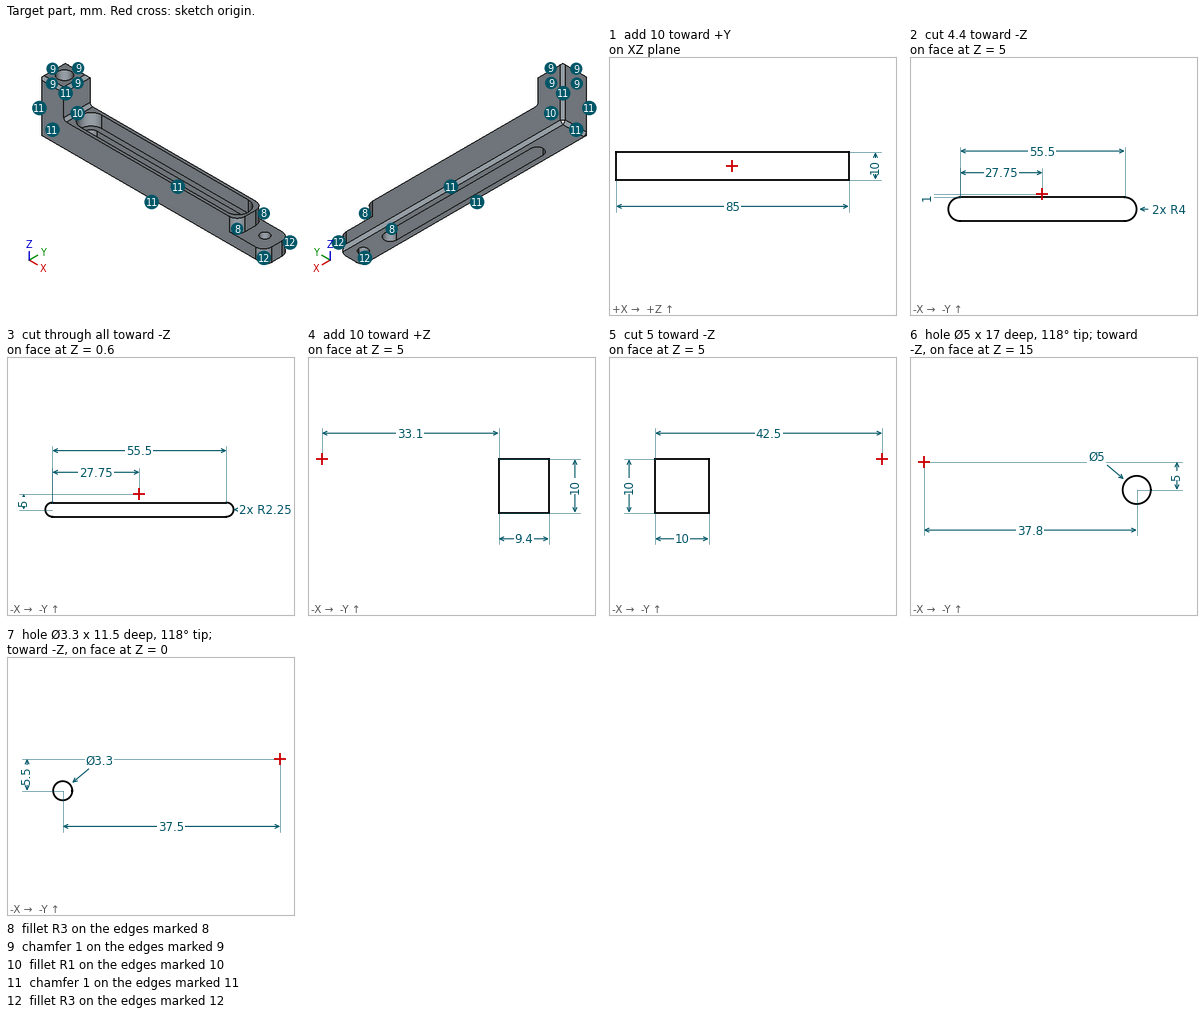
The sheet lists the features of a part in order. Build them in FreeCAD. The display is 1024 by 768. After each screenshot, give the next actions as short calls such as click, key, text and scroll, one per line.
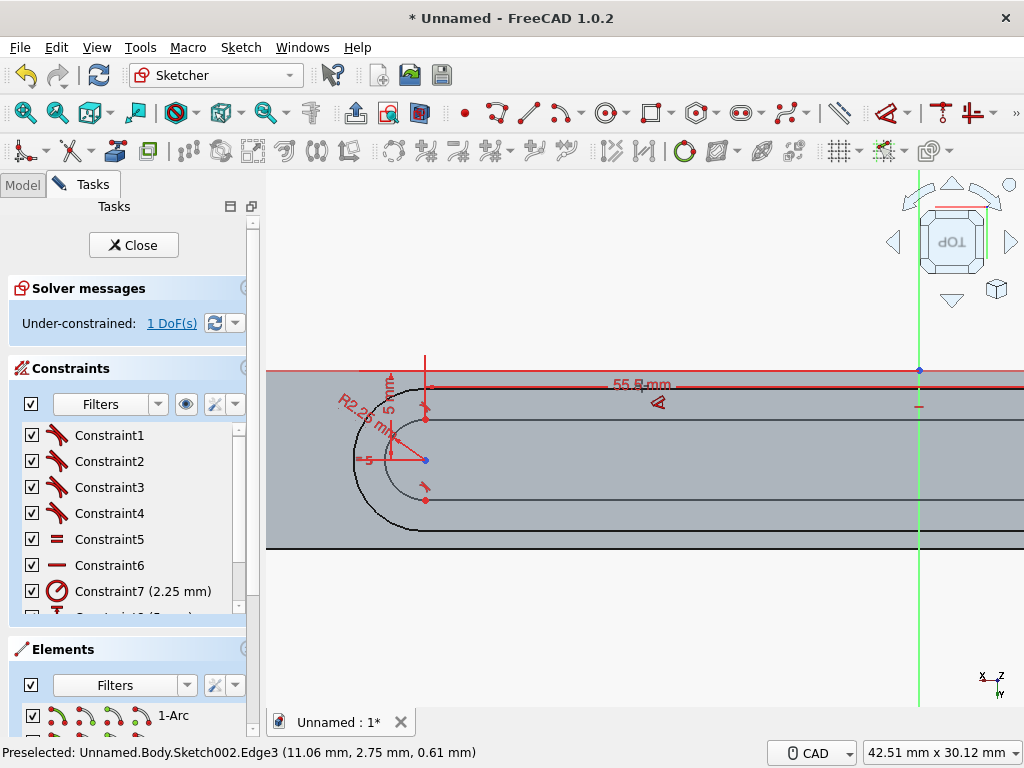
click(425, 420)
click(642, 337)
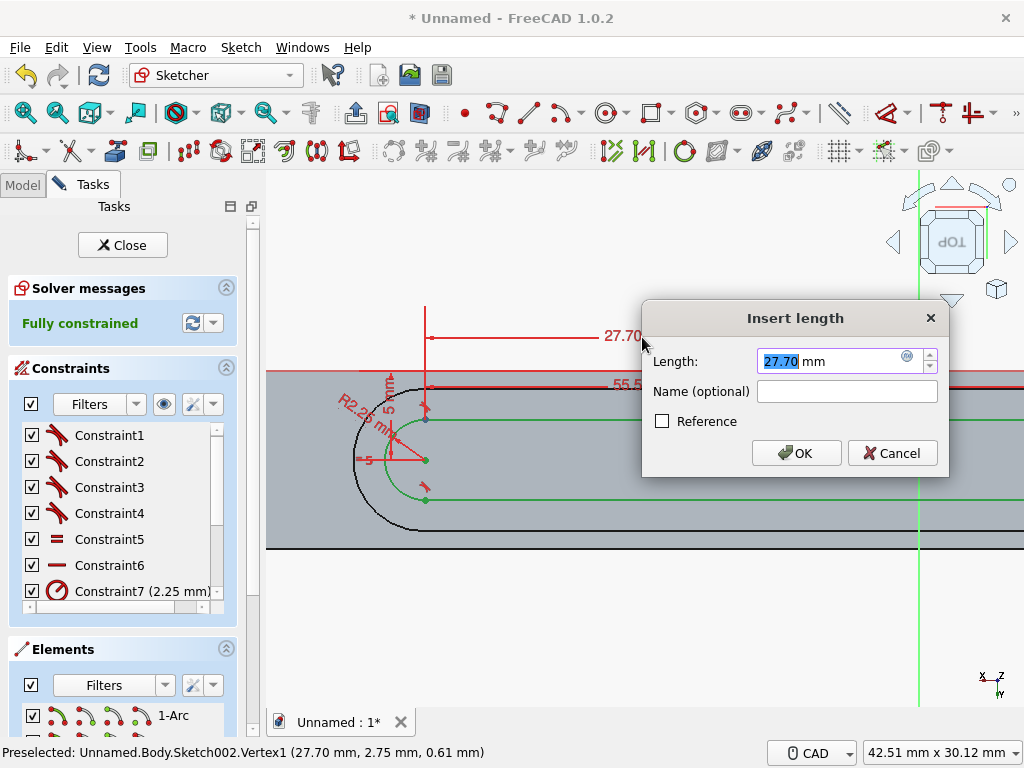
text(27.75)
key(Return)
key(Escape)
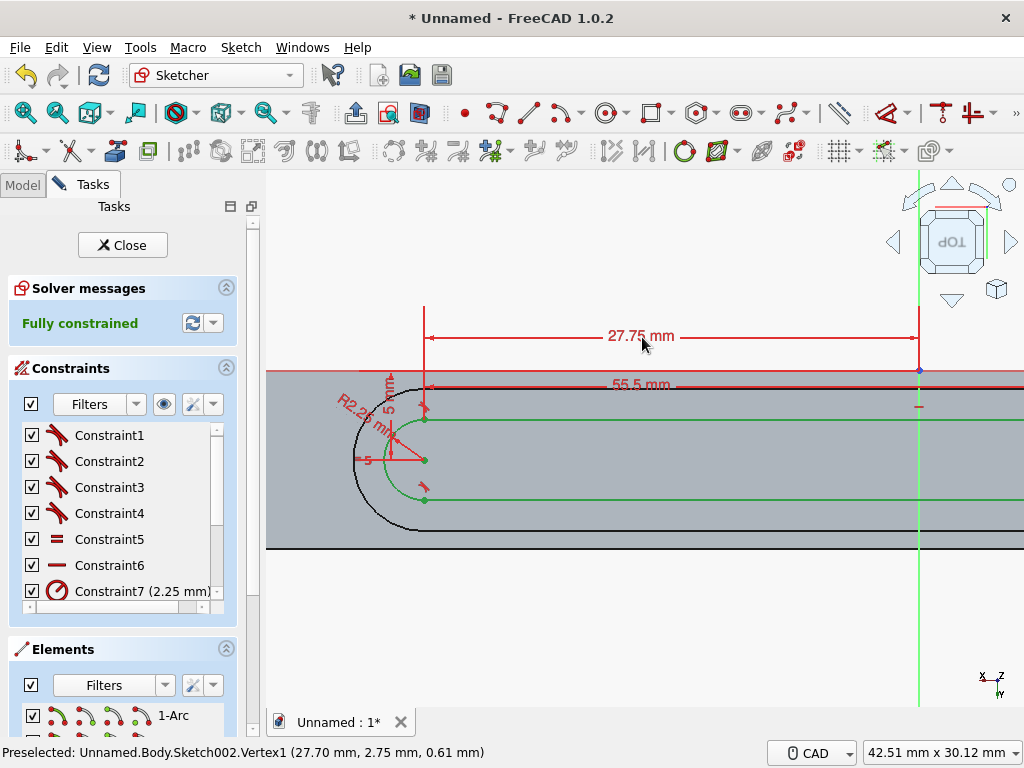
click(123, 245)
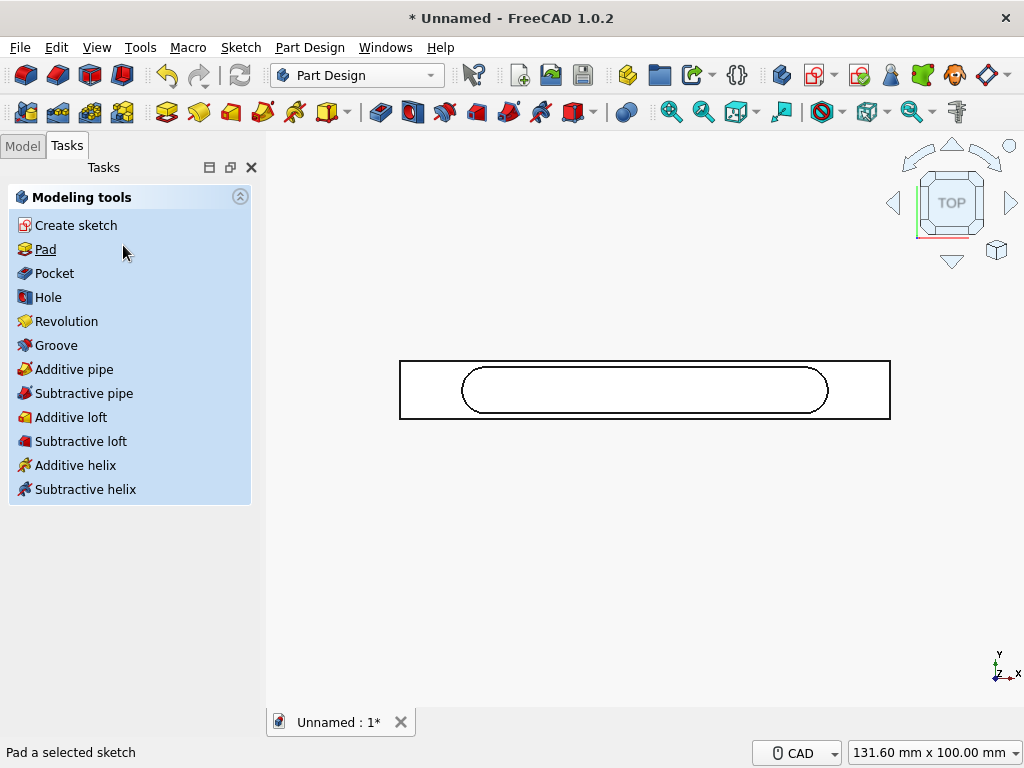
click(382, 112)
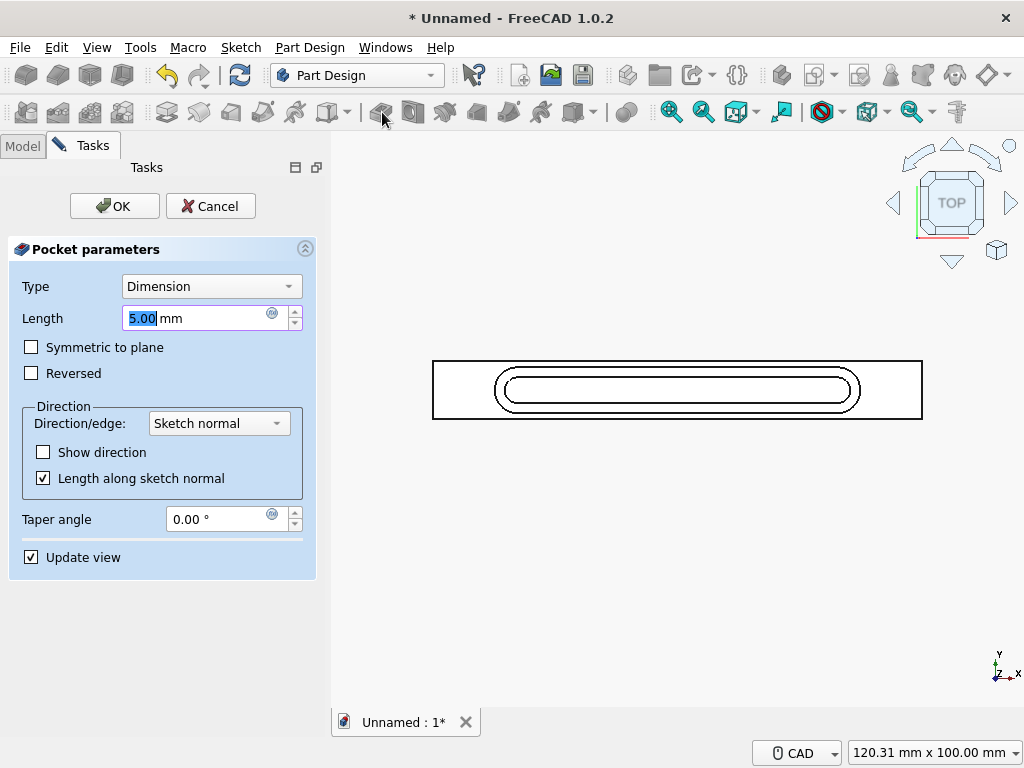
click(212, 286)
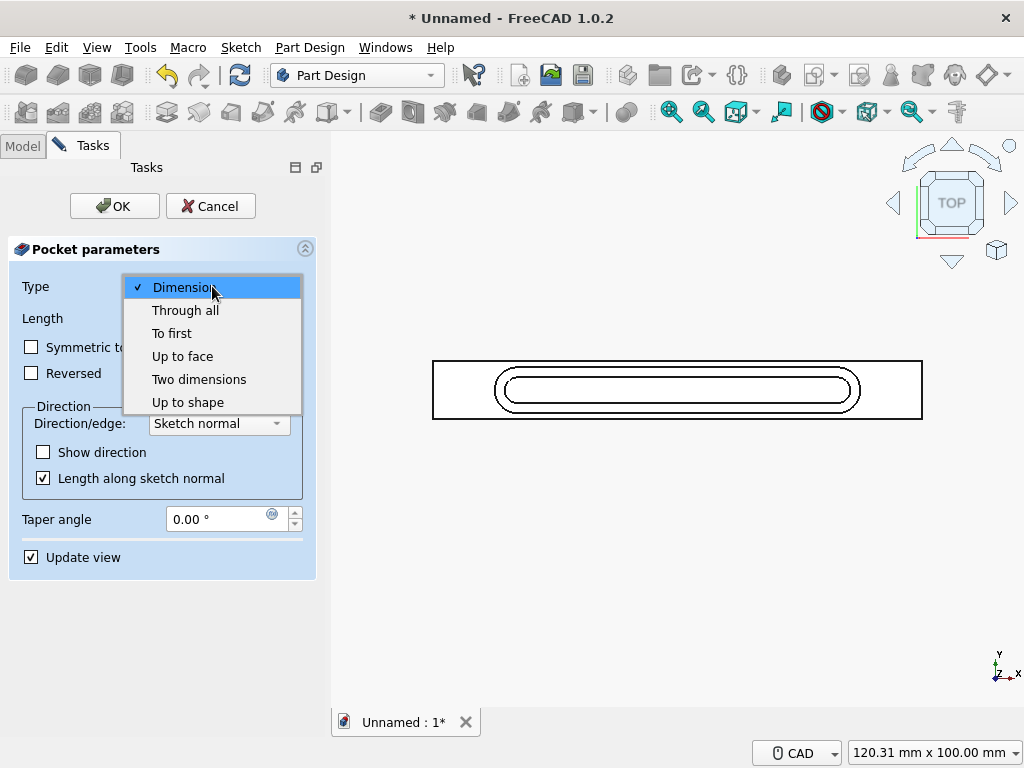
click(212, 310)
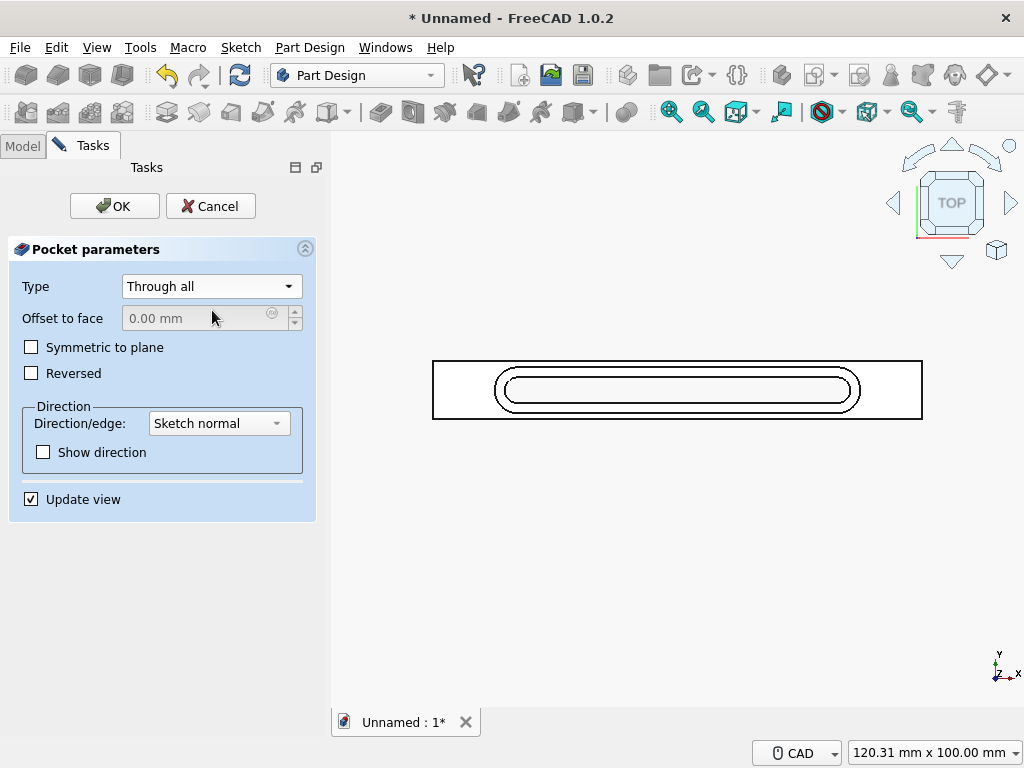
click(115, 206)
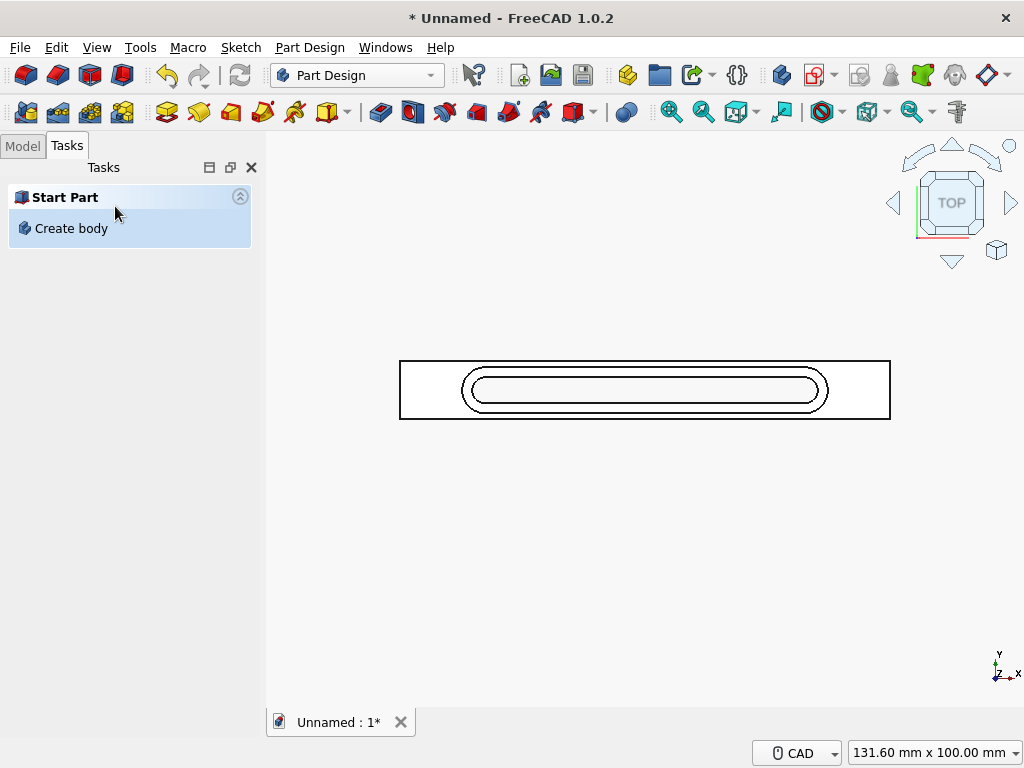
click(855, 389)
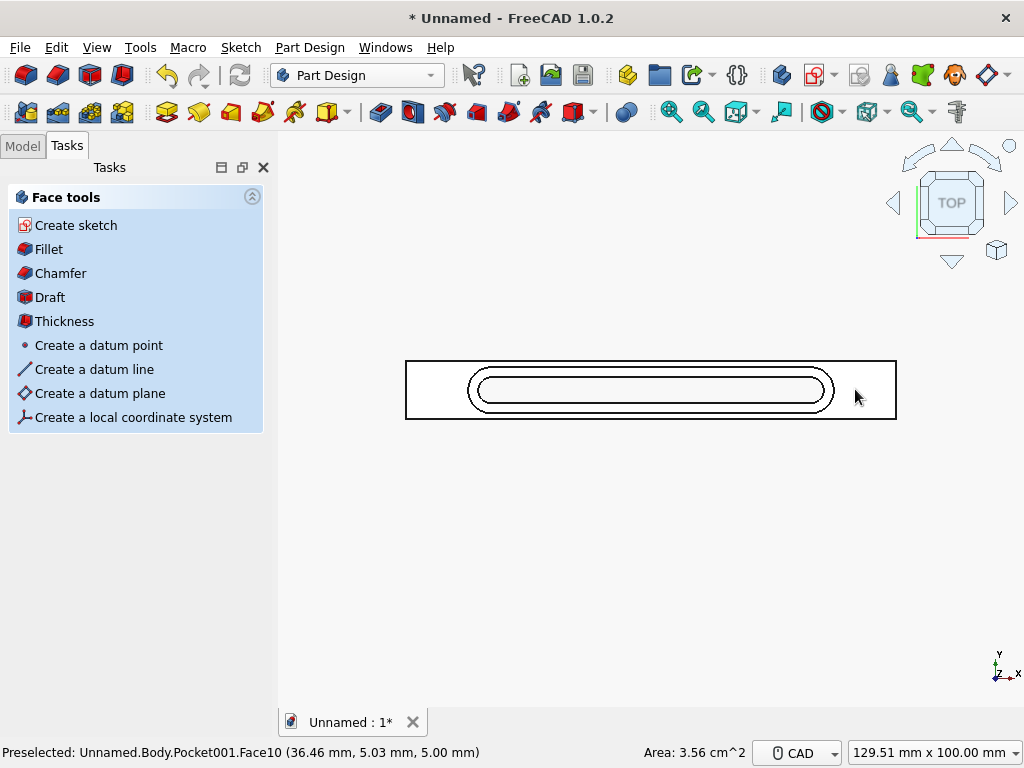
click(814, 76)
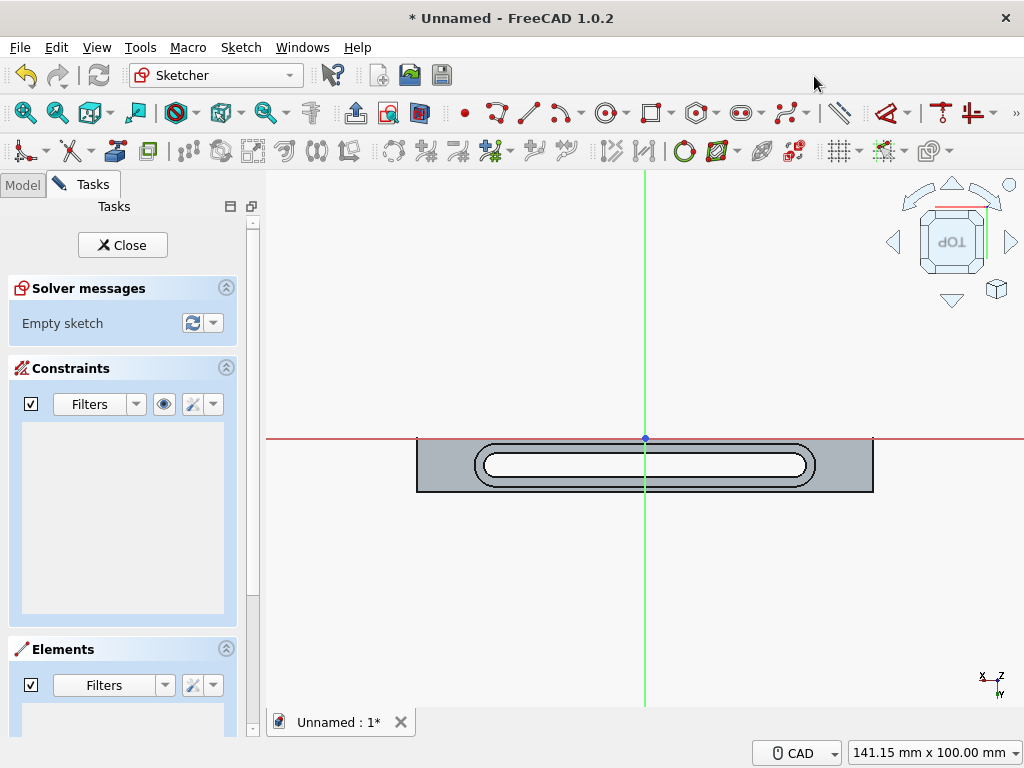
scroll(576, 438, down, 5)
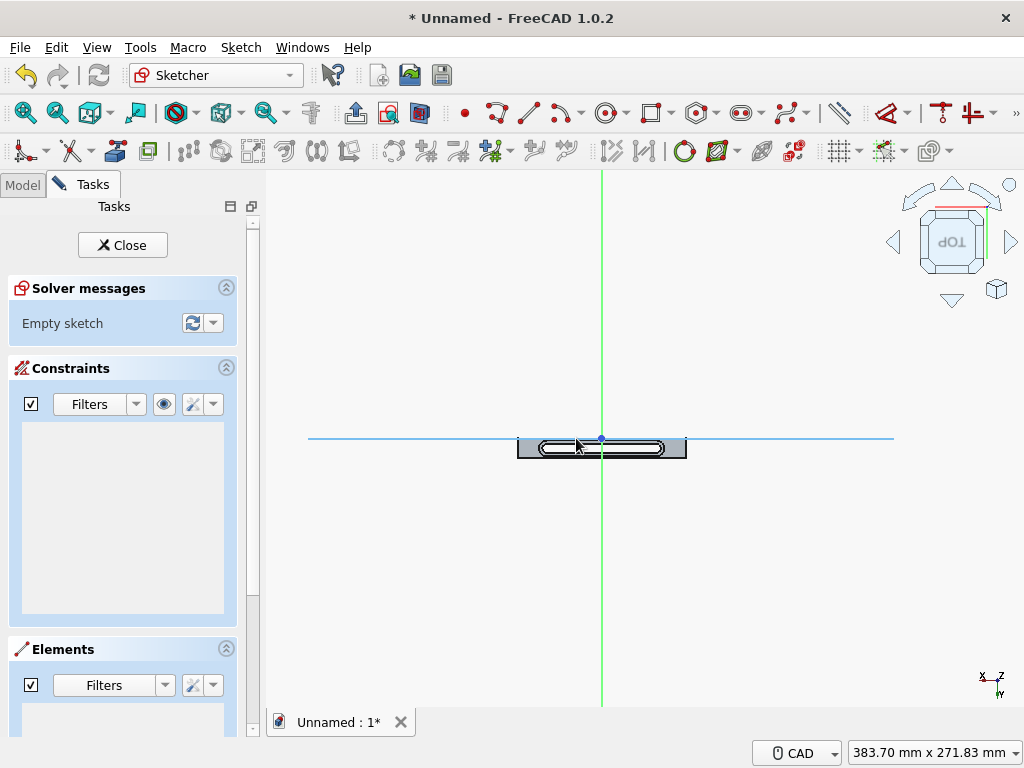
scroll(683, 449, up, 14)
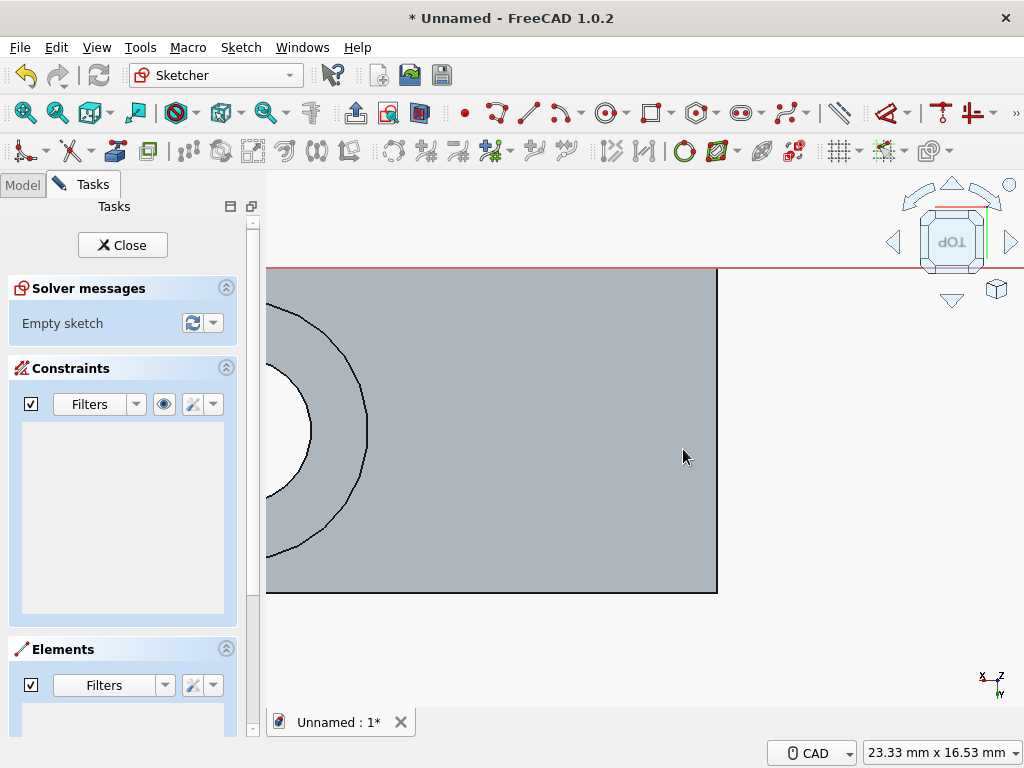
click(652, 114)